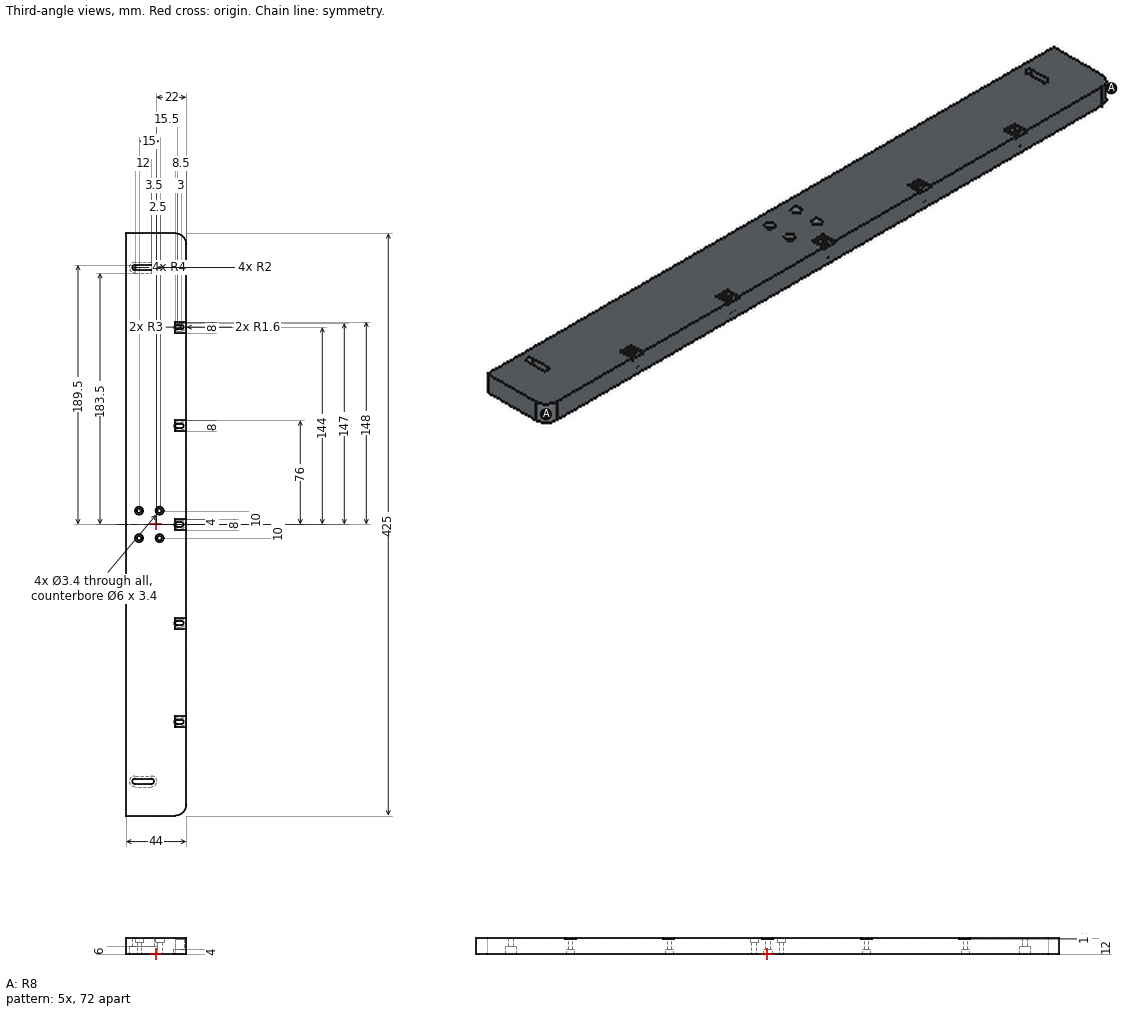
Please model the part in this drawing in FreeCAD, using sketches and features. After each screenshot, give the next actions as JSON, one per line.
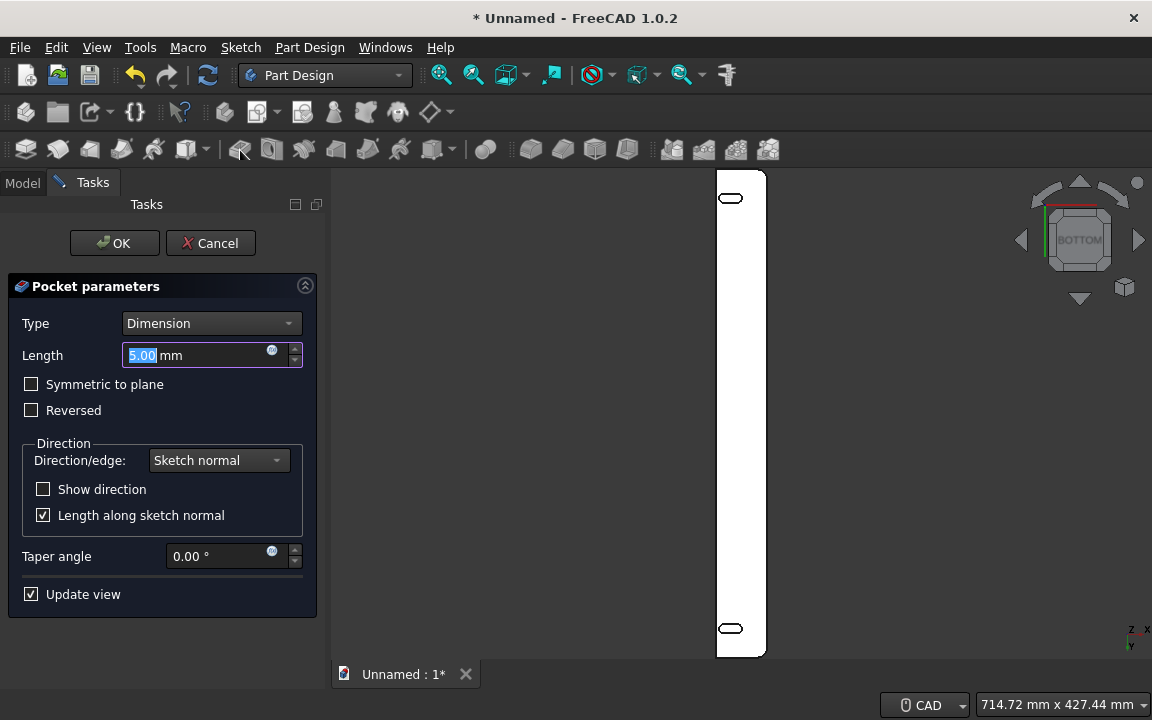
{"action": "type", "text": "6"}
{"action": "key", "text": "Tab"}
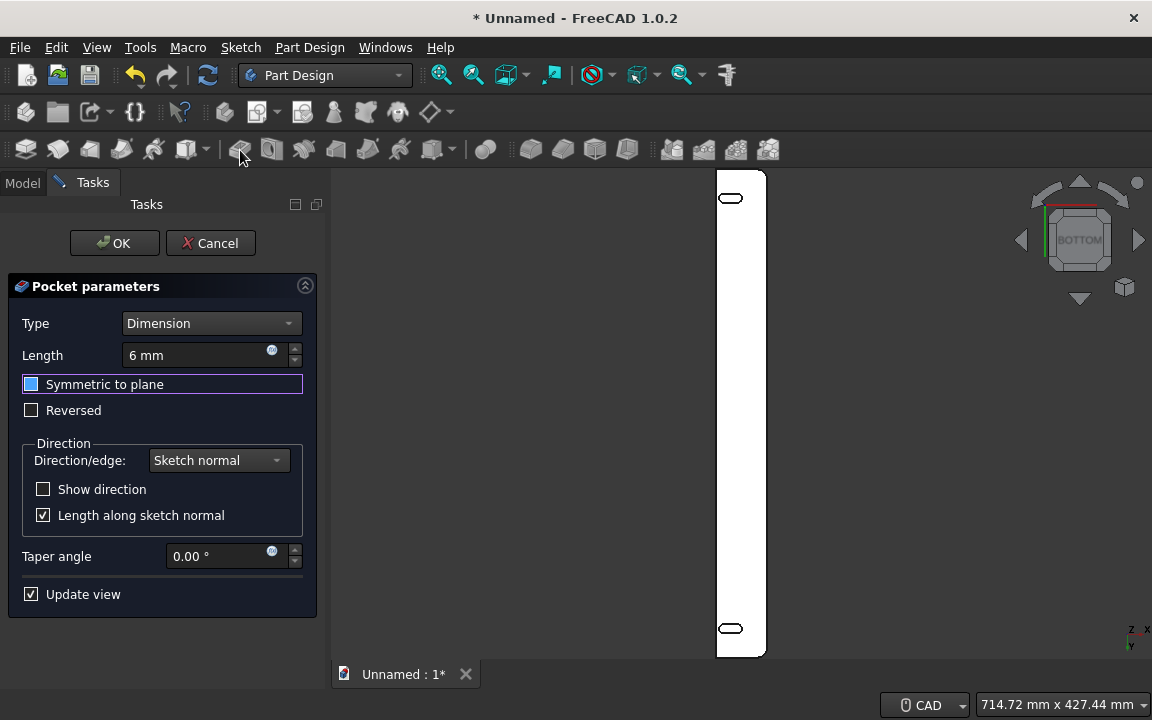
{"action": "left_click", "coordinate": [115, 243]}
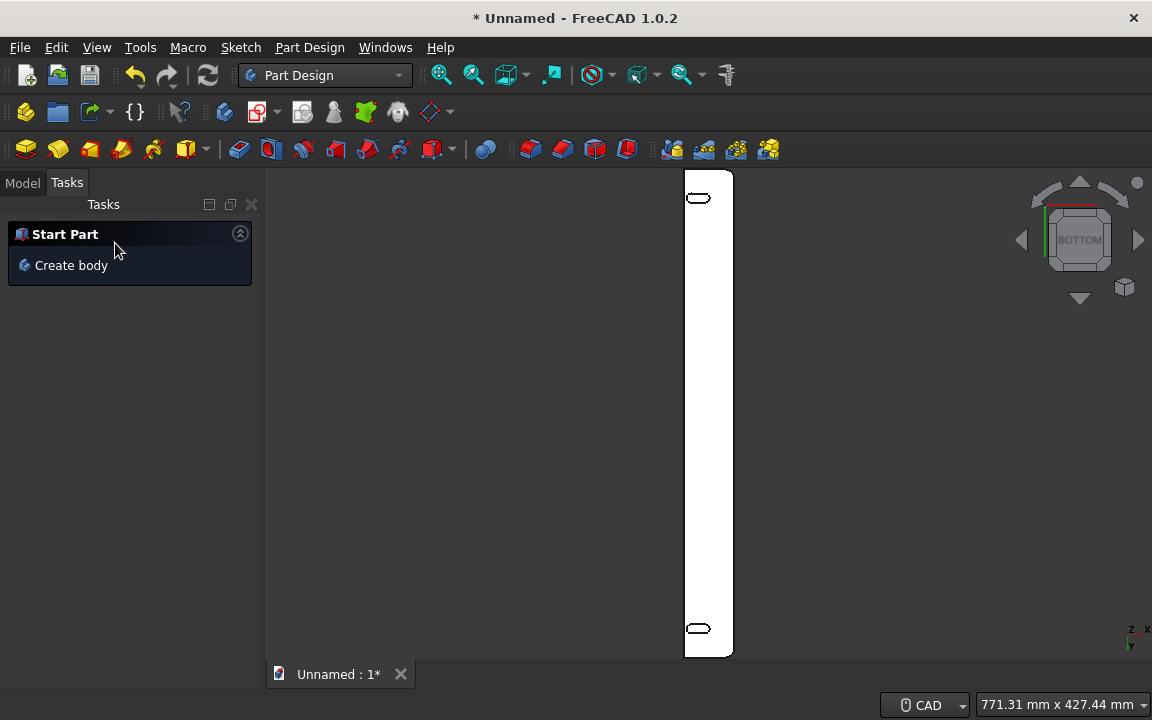
{"action": "left_click", "coordinate": [258, 112]}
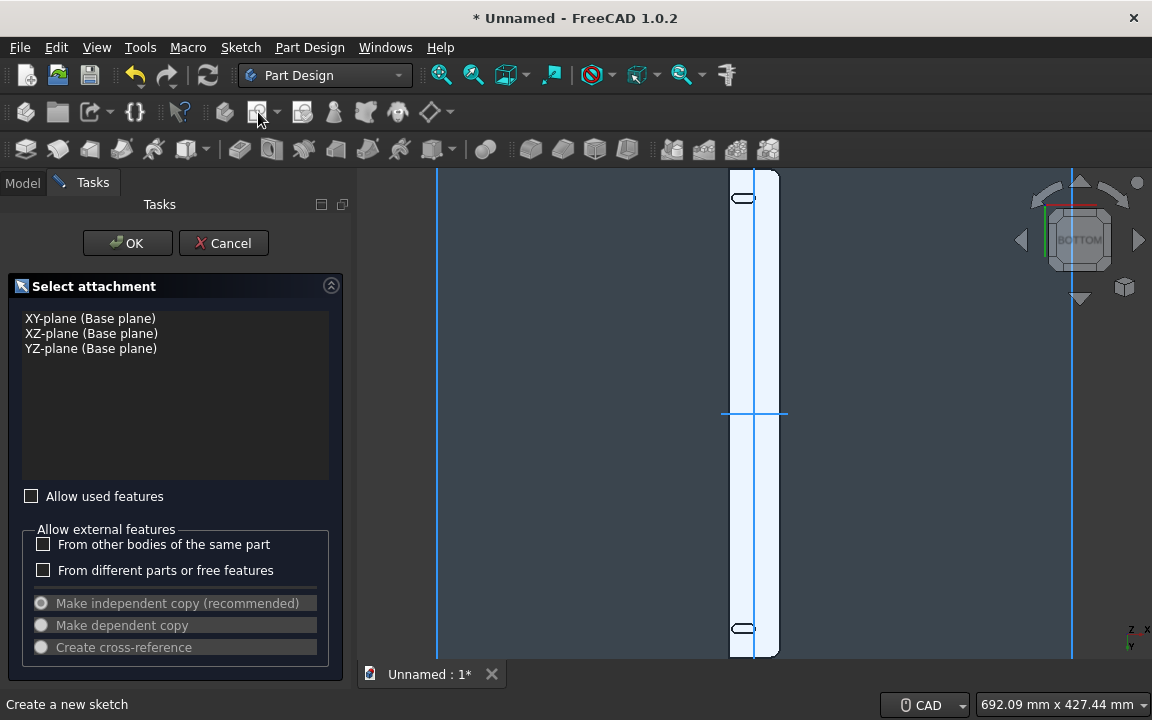
{"action": "left_click", "coordinate": [82, 318]}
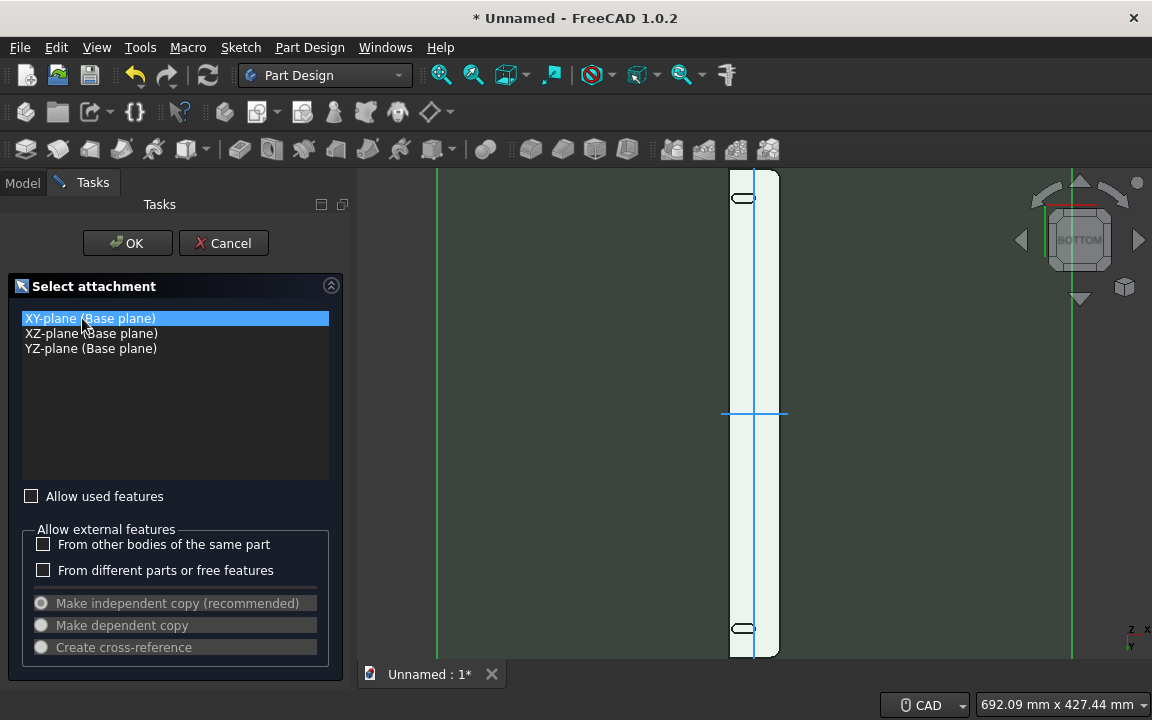
{"action": "left_click", "coordinate": [128, 243]}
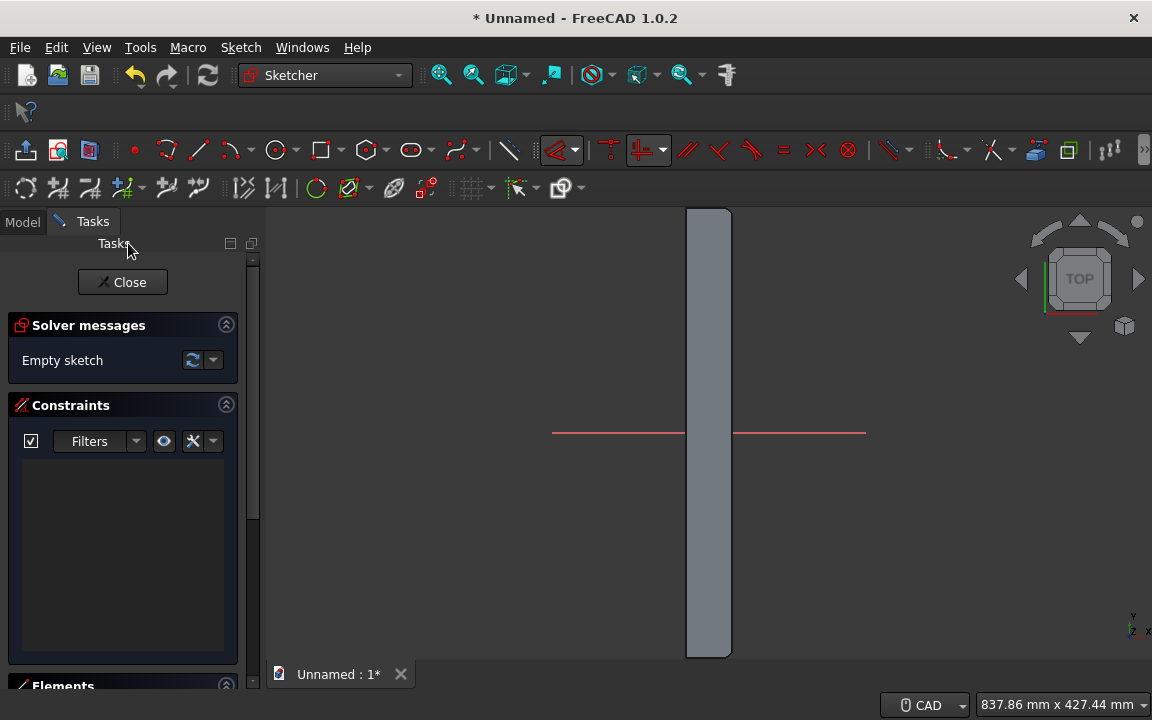
{"action": "left_click", "coordinate": [90, 150]}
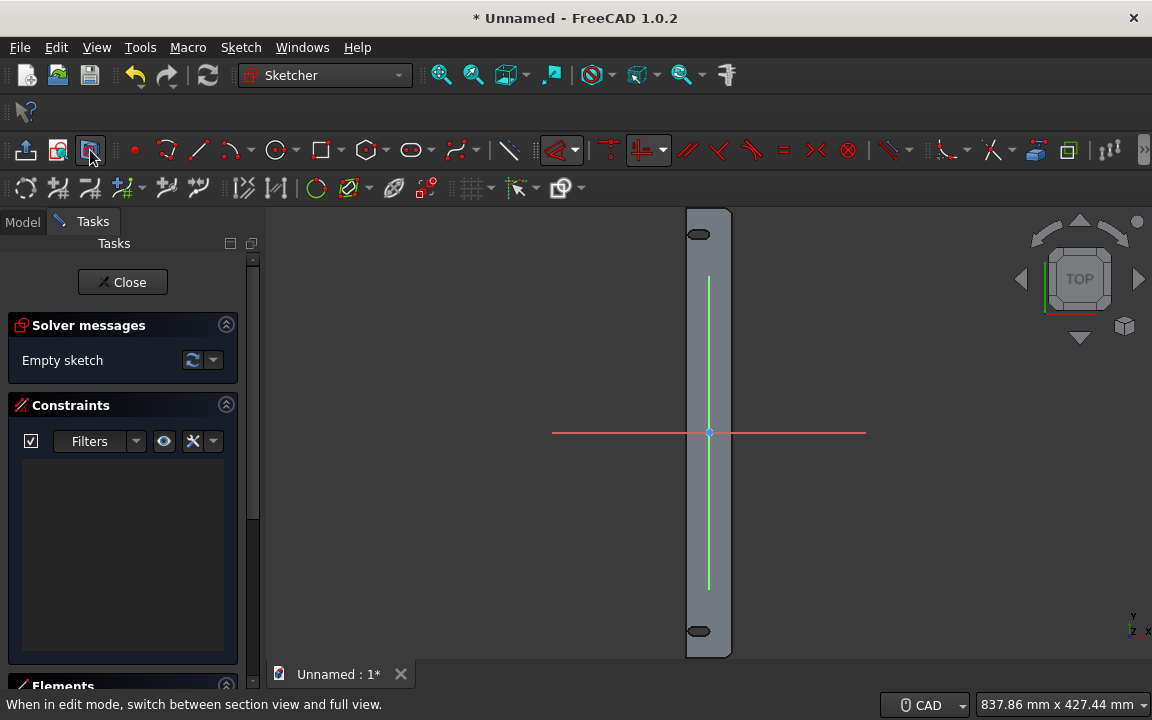
{"action": "scroll", "coordinate": [520, 433], "scroll_direction": "down", "scroll_amount": 2}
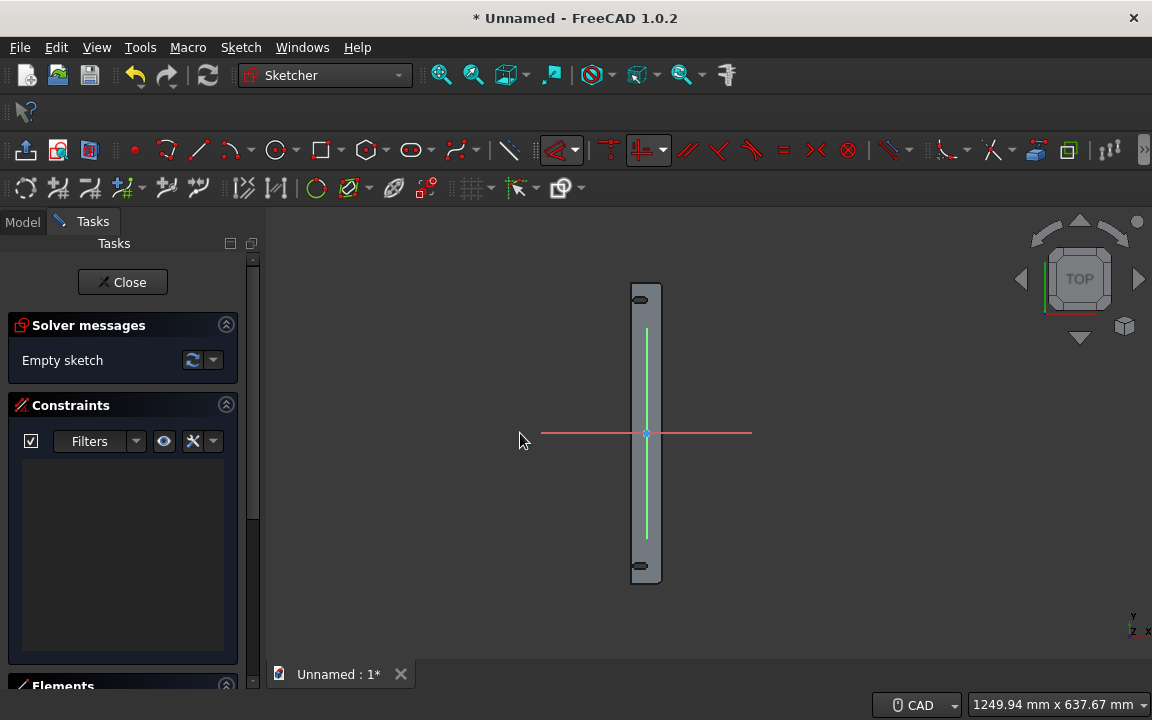
{"action": "key", "text": "g s"}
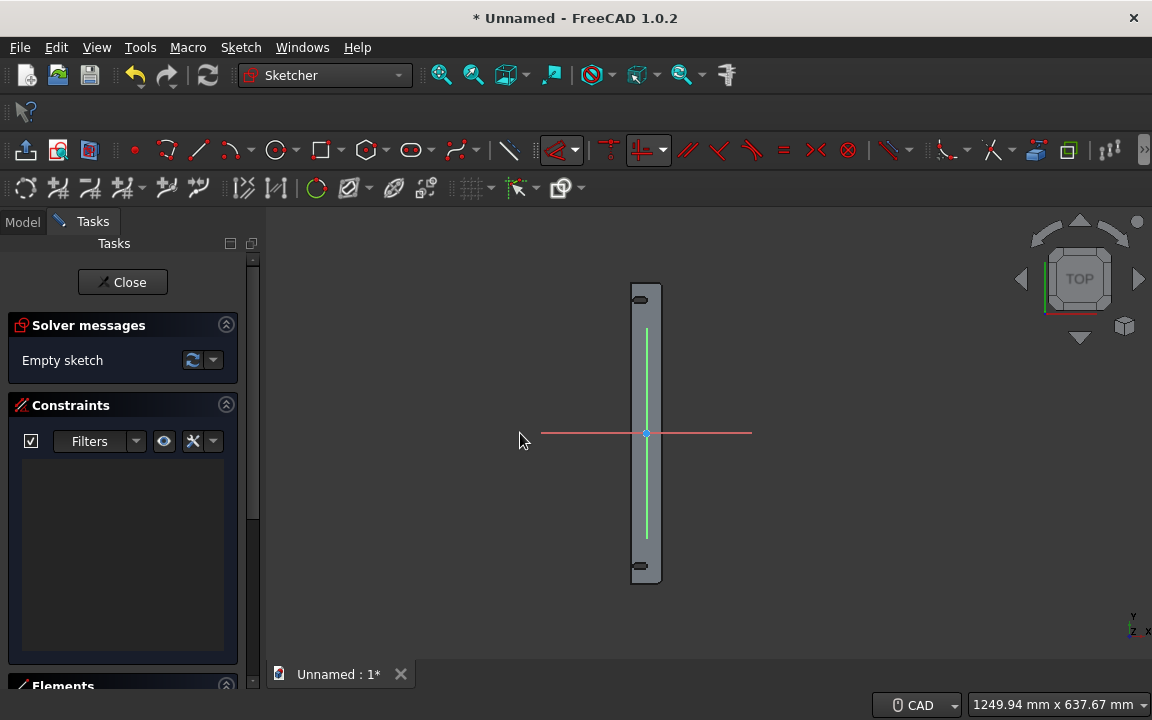
{"action": "scroll", "coordinate": [636, 300], "scroll_direction": "up", "scroll_amount": 14}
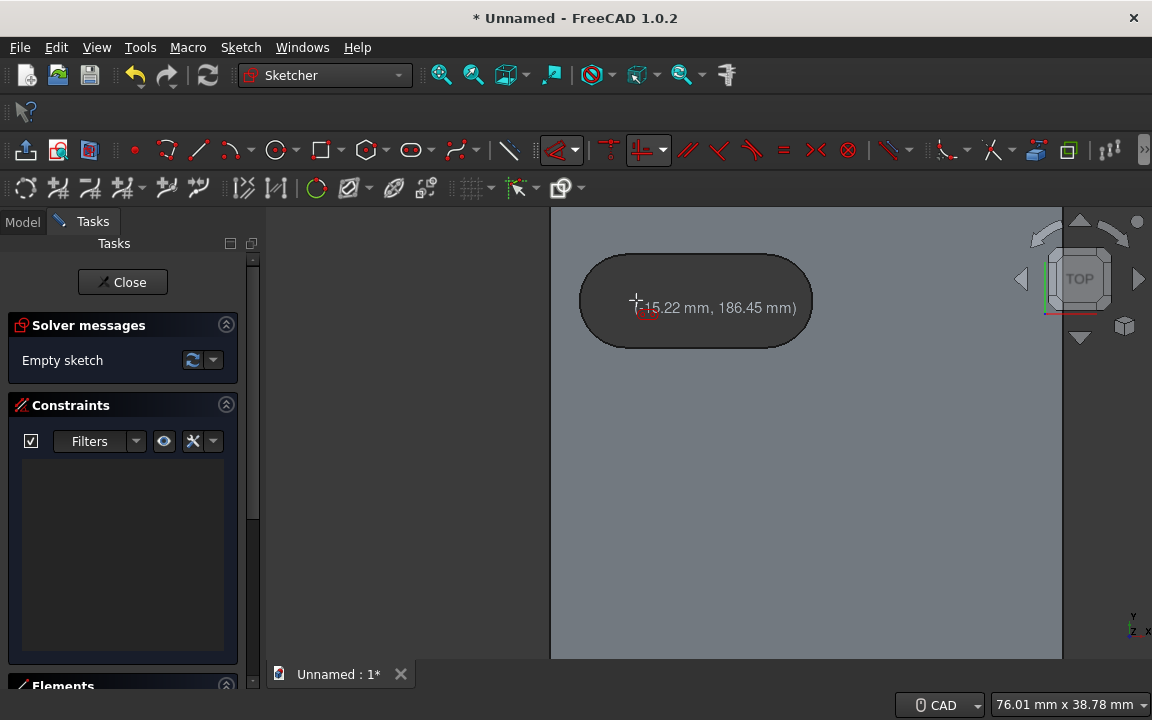
{"action": "scroll", "coordinate": [636, 300], "scroll_direction": "down", "scroll_amount": 14}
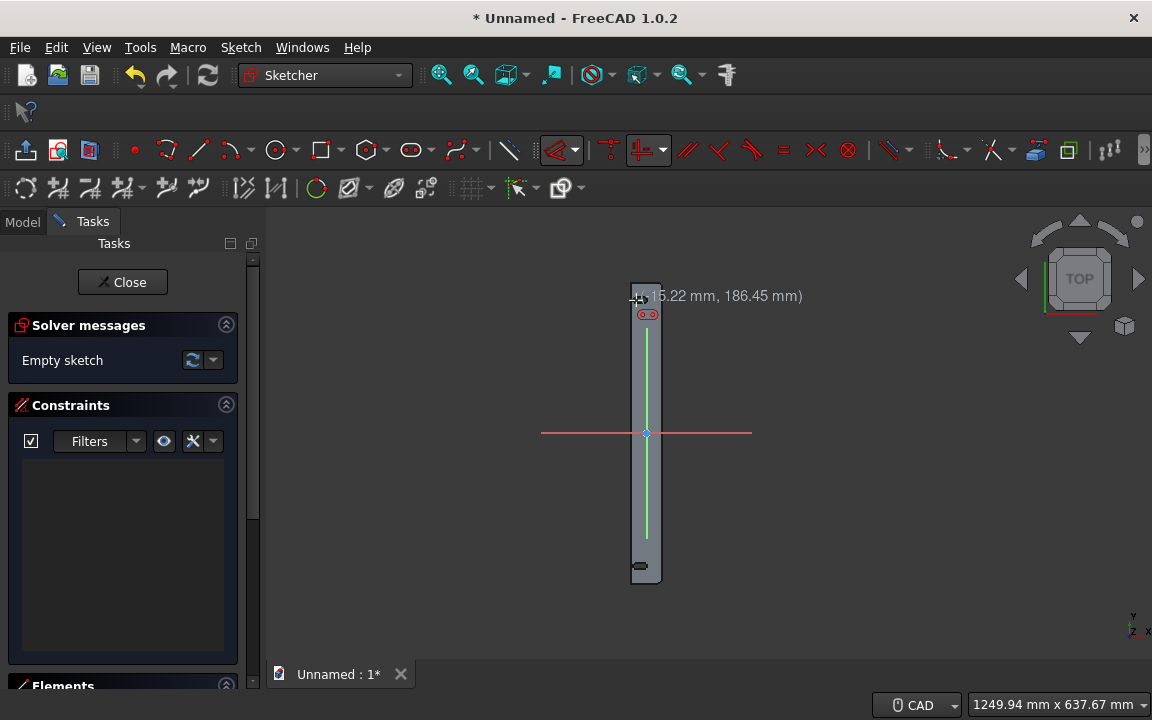
{"action": "scroll", "coordinate": [636, 300], "scroll_direction": "up", "scroll_amount": 2}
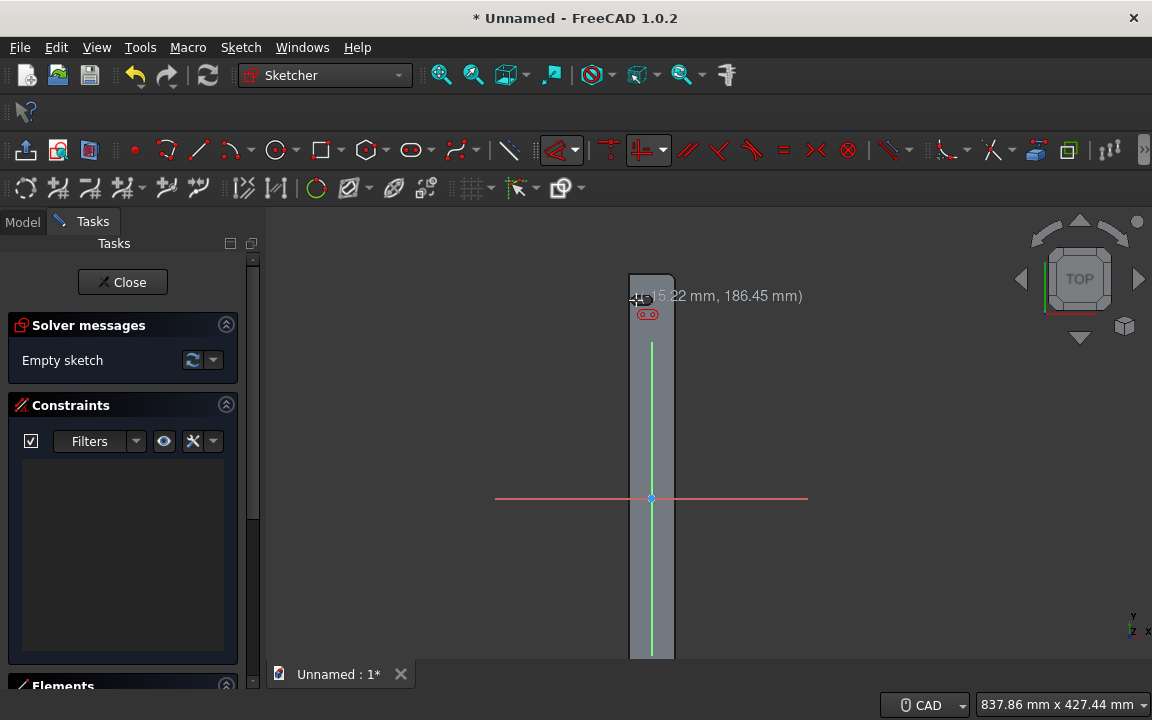
{"action": "left_click", "coordinate": [635, 300]}